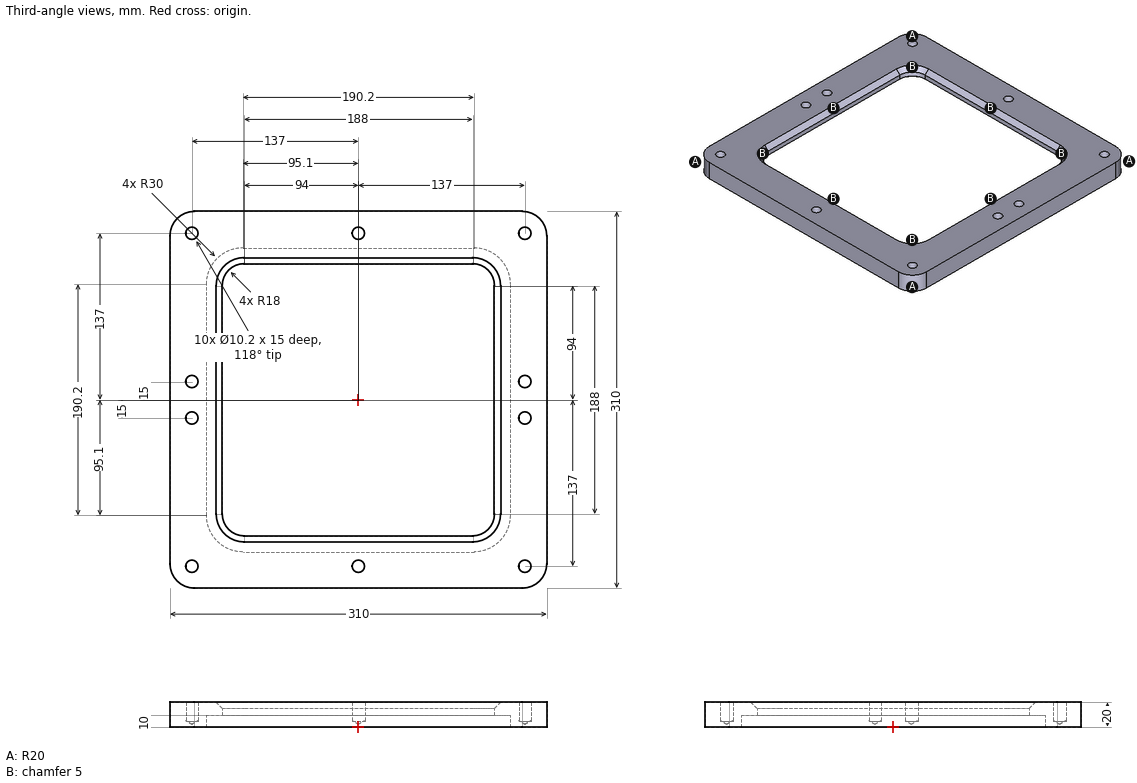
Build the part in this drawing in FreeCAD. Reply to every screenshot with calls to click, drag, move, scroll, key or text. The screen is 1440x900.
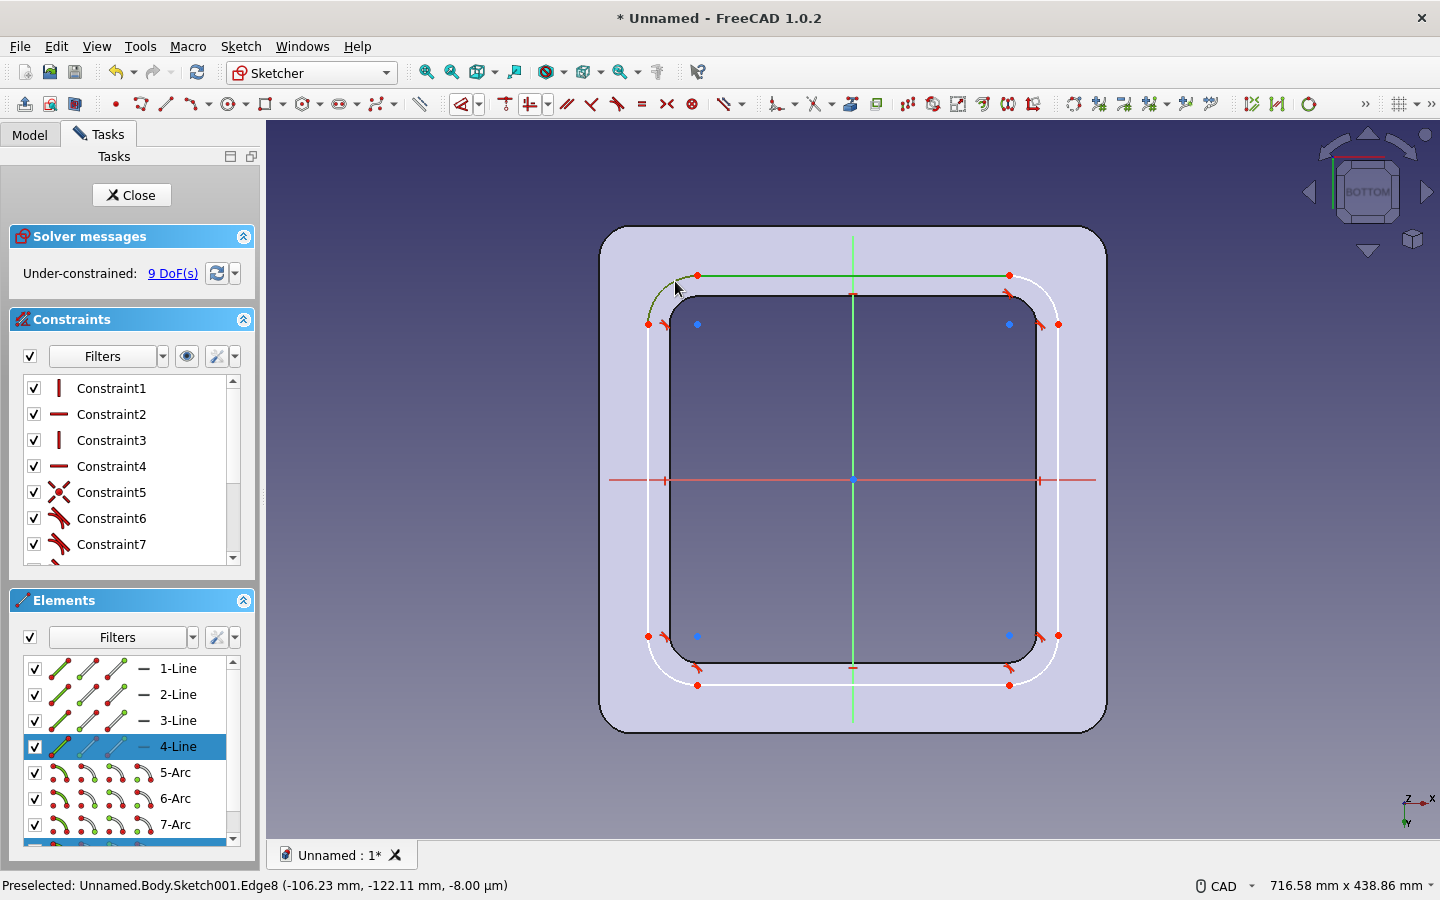
click(617, 104)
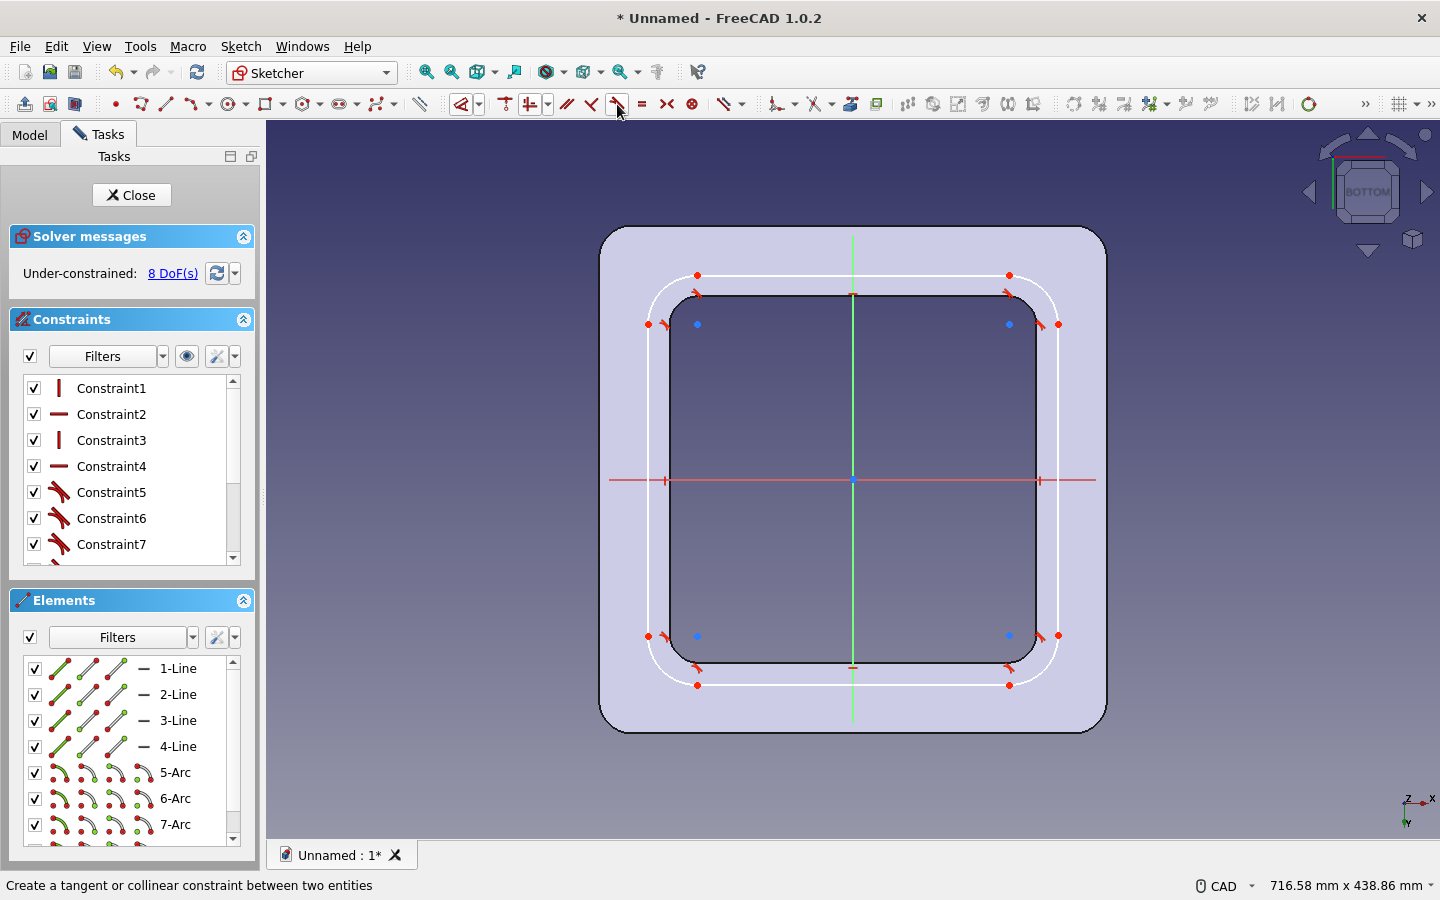
click(653, 658)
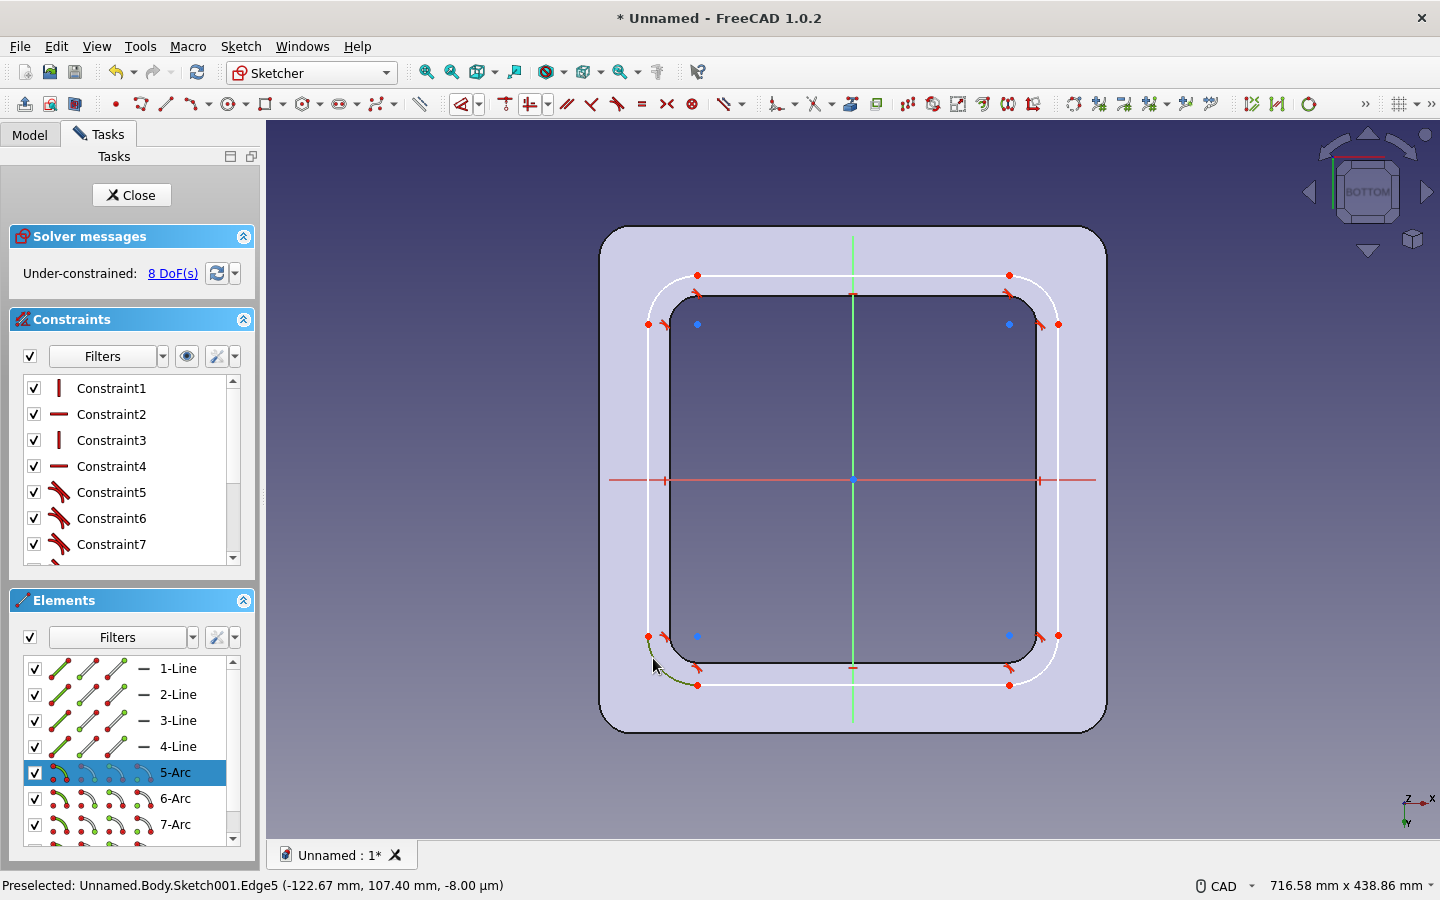
click(1031, 680)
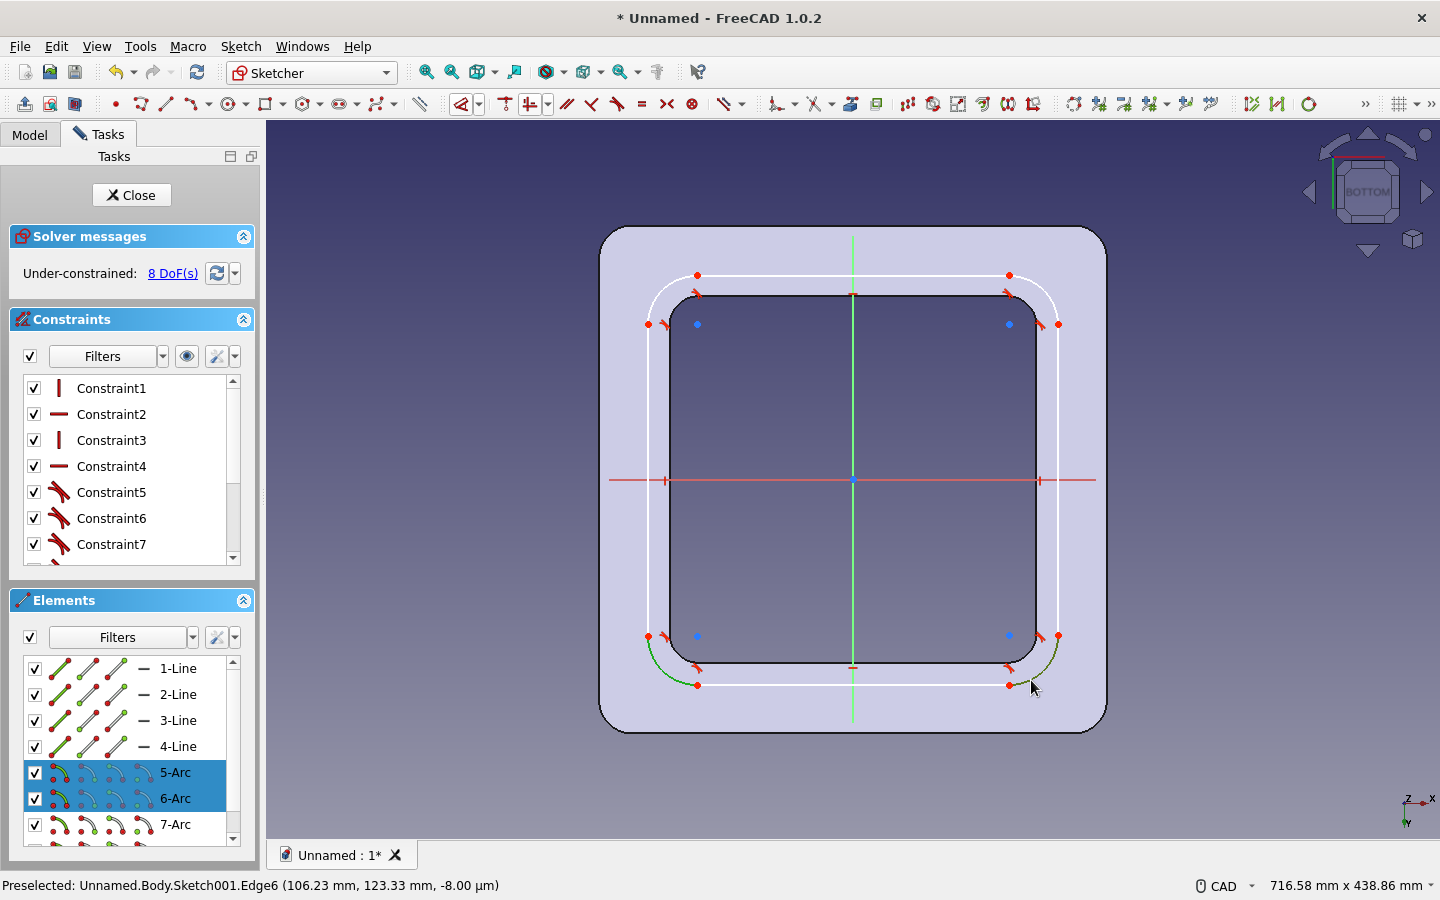
click(1053, 303)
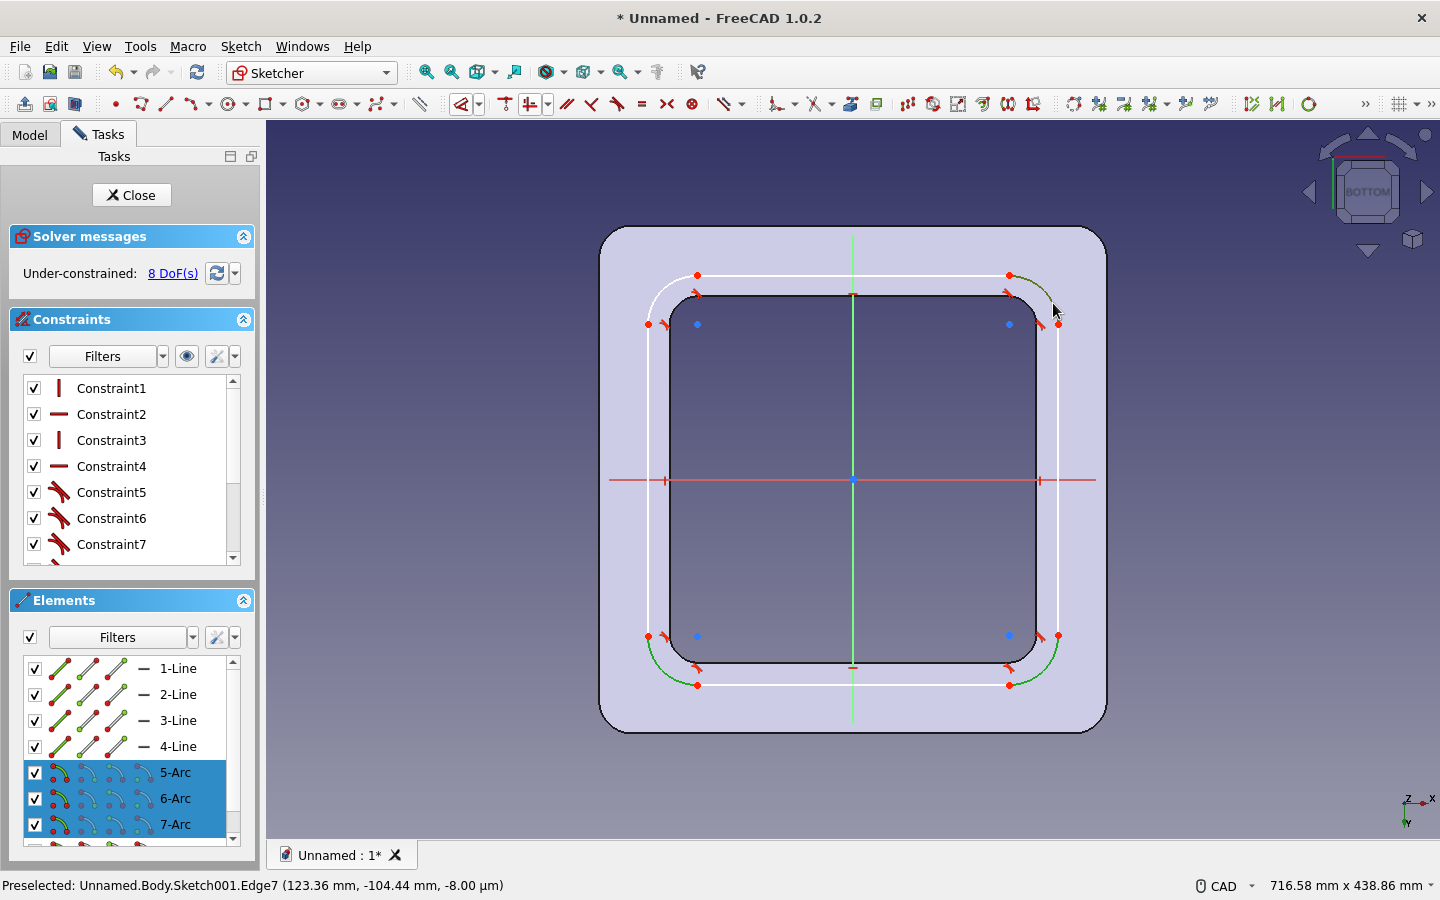
click(675, 281)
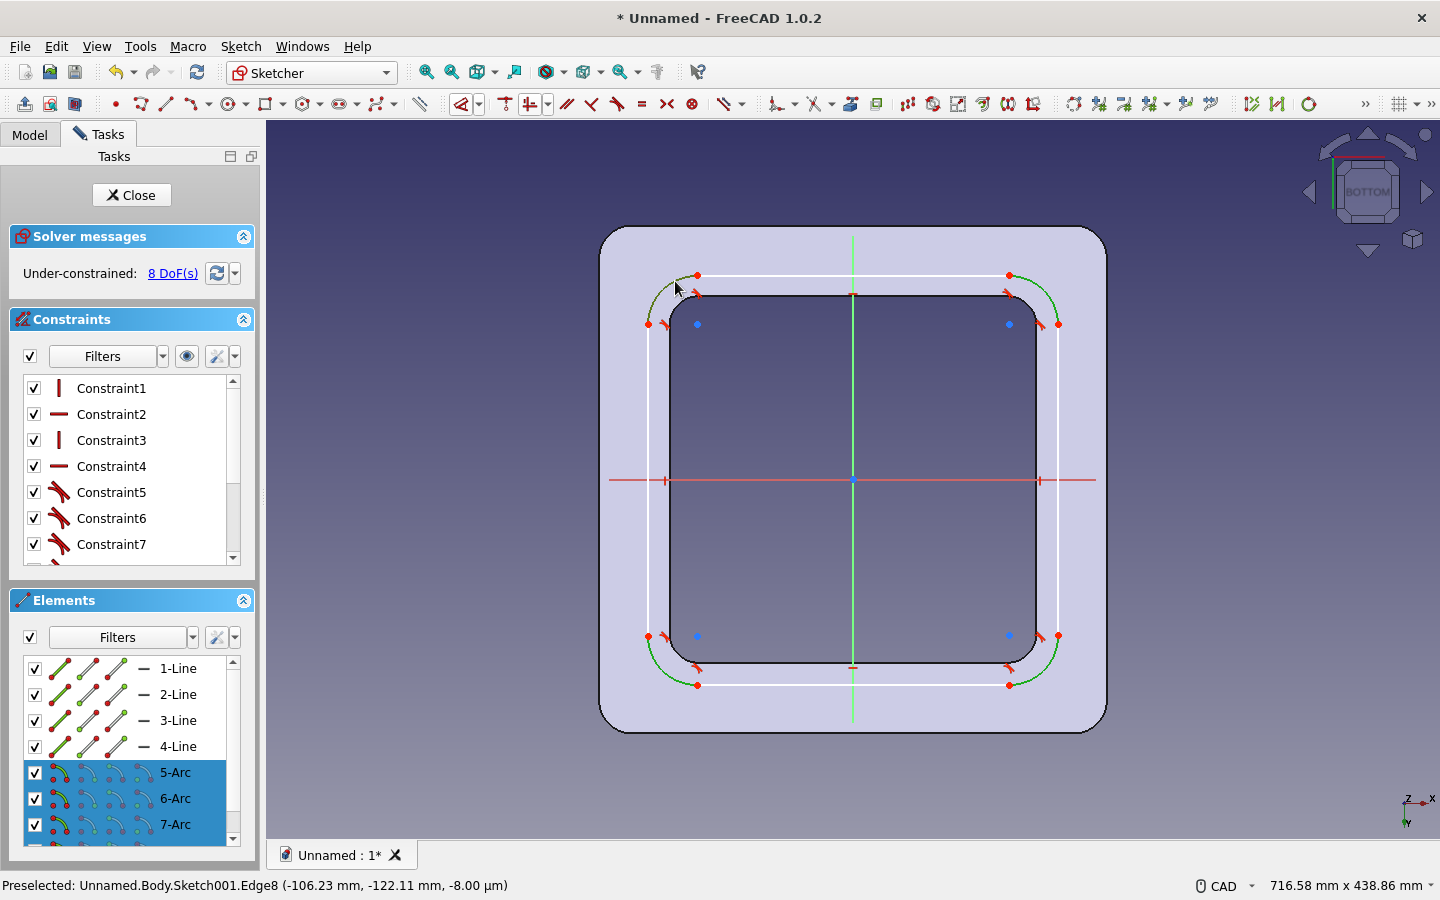
click(642, 104)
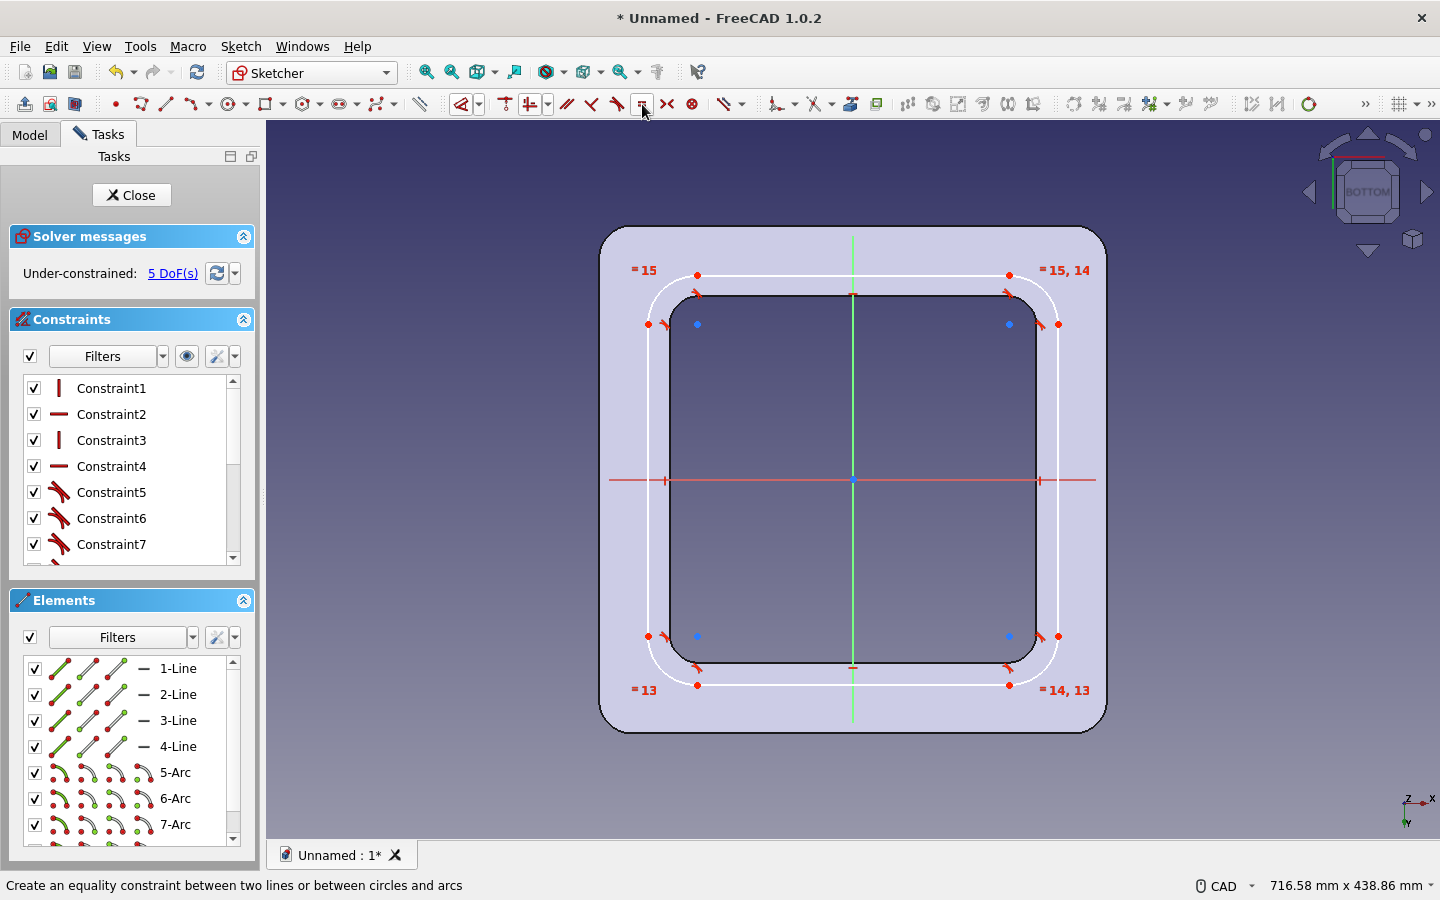
click(653, 658)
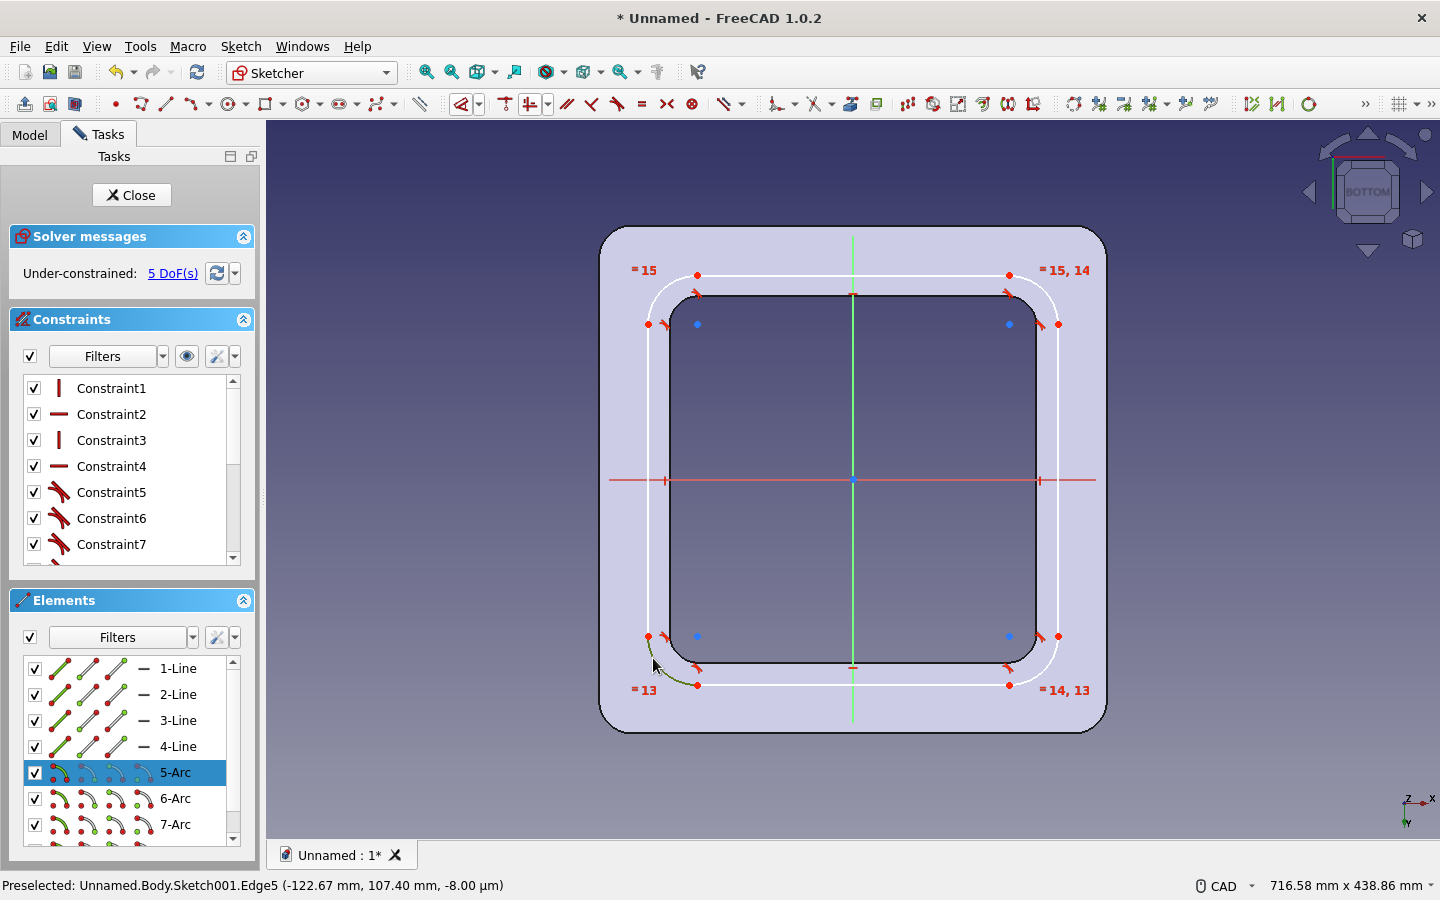
key(k)
key(r)